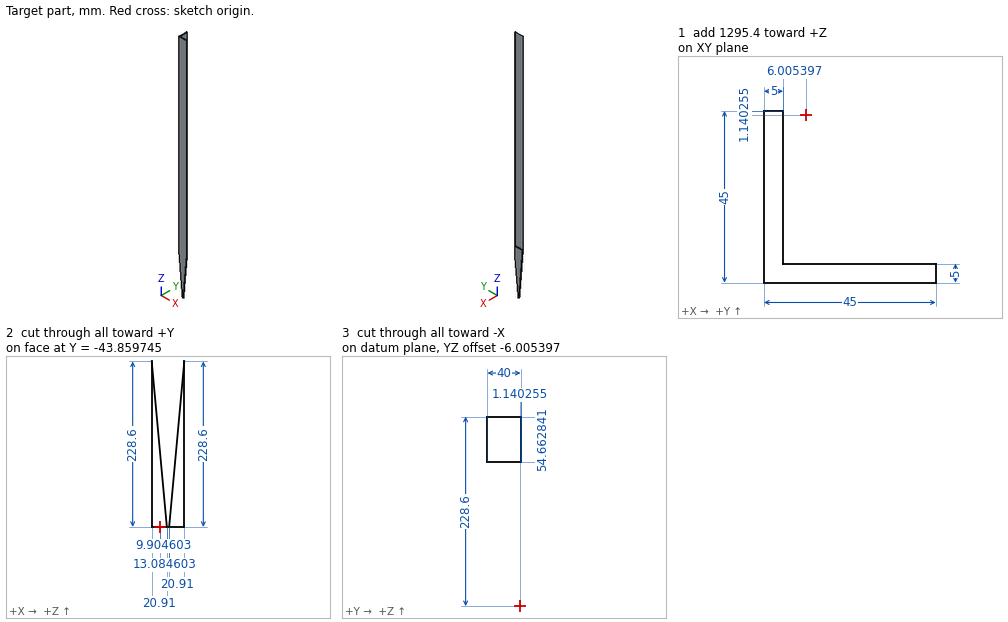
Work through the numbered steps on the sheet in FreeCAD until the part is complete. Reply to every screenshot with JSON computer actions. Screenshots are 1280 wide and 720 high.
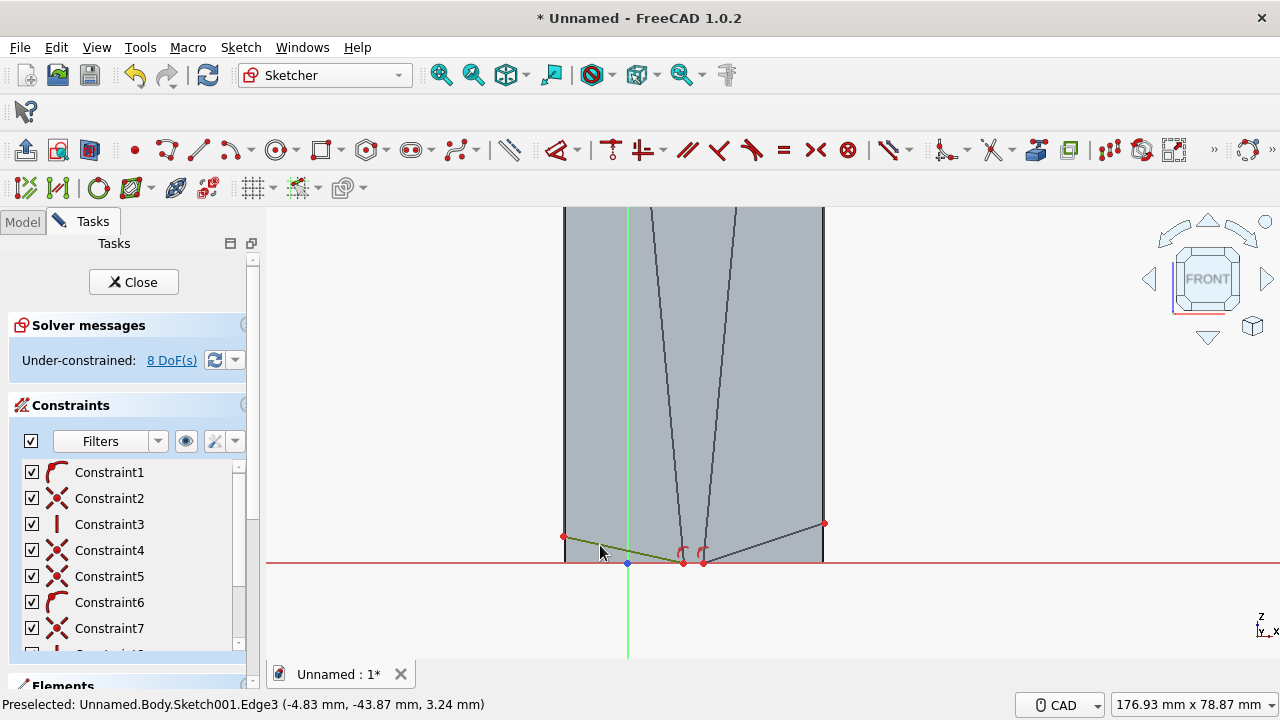
{"action": "key", "text": "h"}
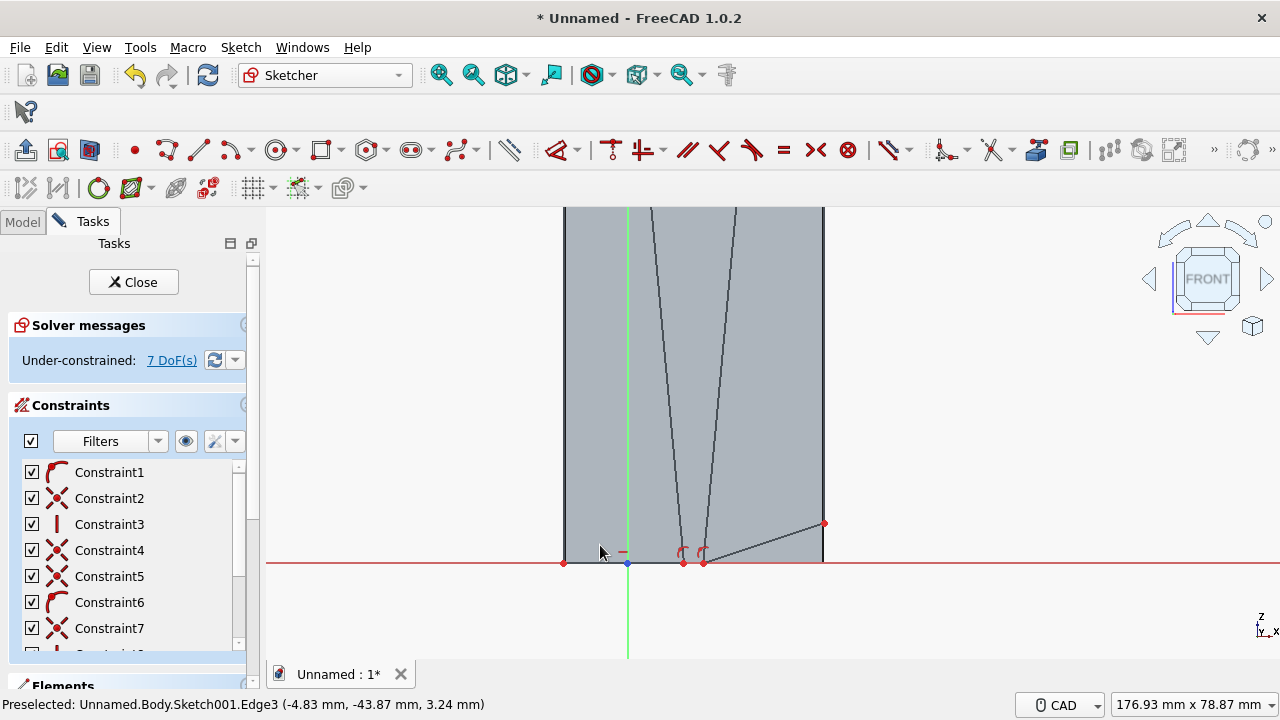
{"action": "left_click", "coordinate": [739, 551]}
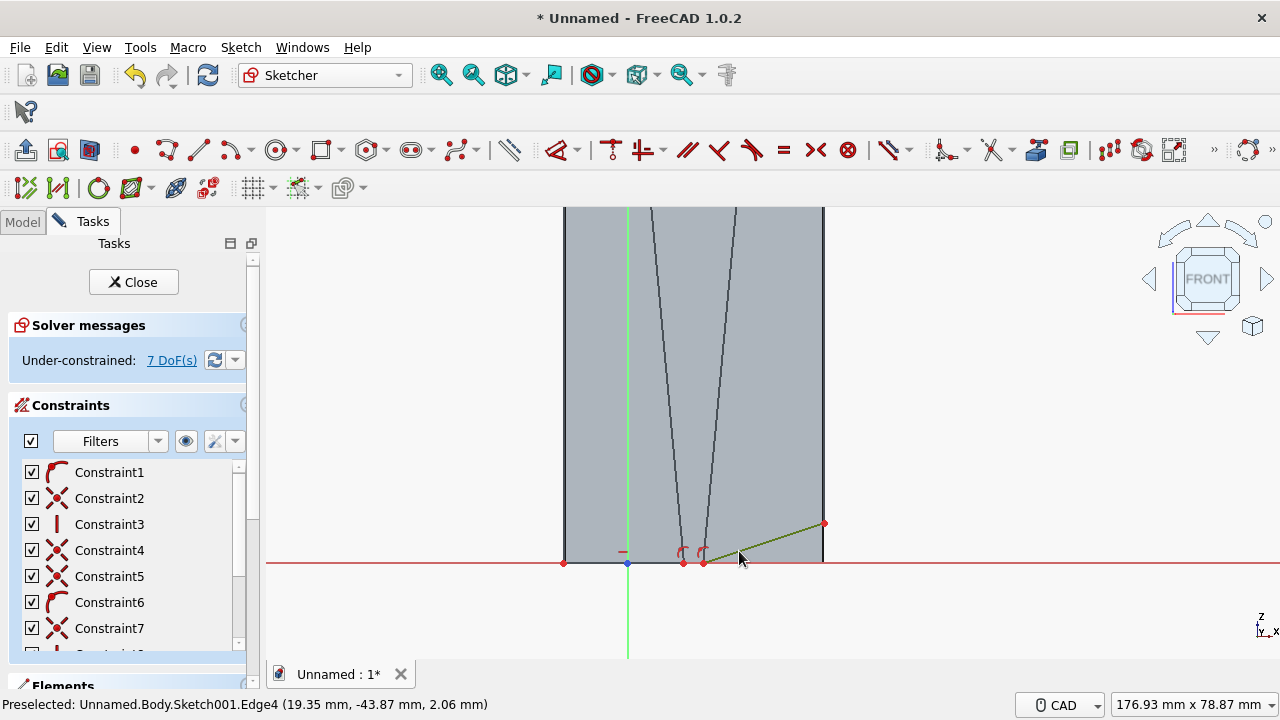
{"action": "key", "text": "h"}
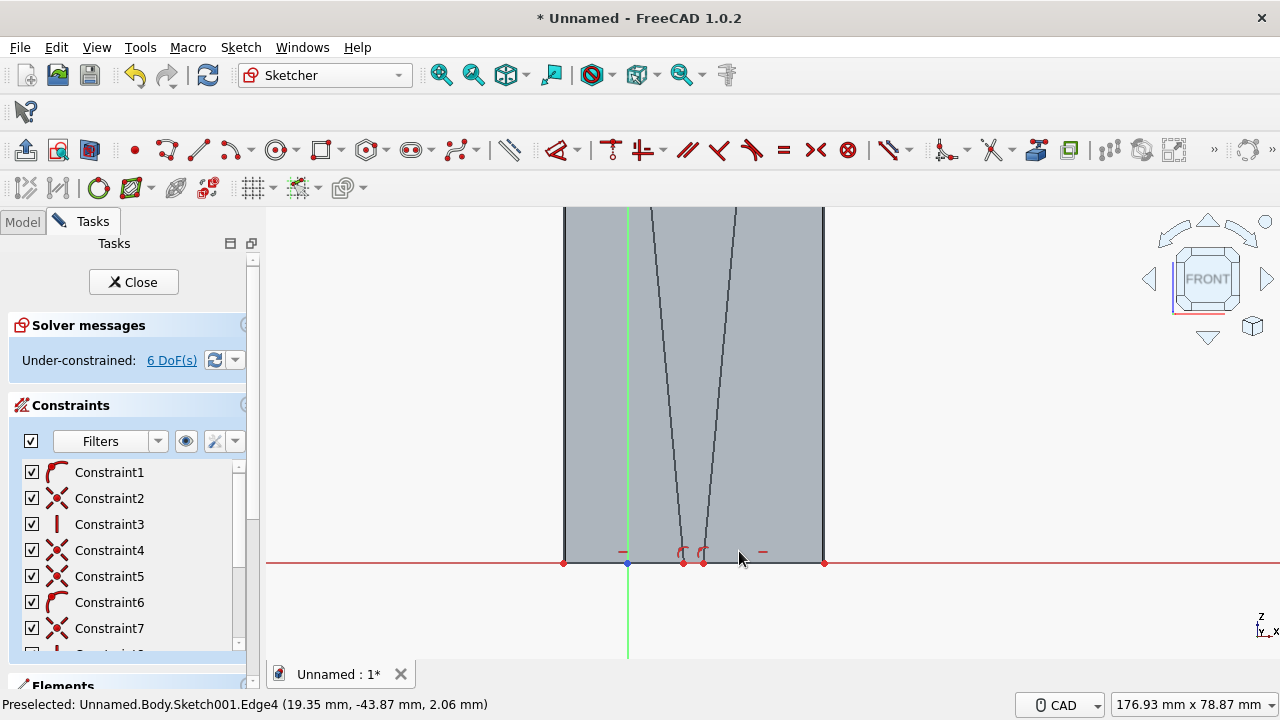
{"action": "left_click", "coordinate": [556, 150]}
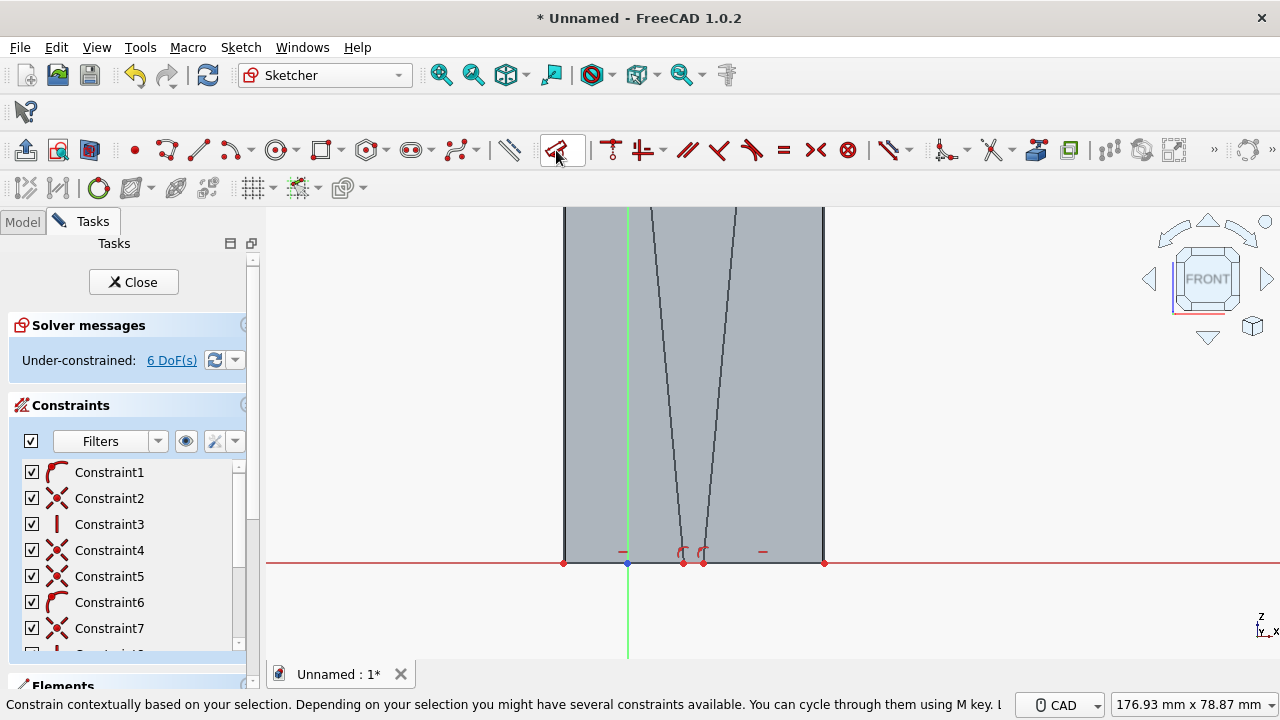
{"action": "scroll", "coordinate": [707, 566], "scroll_direction": "down", "scroll_amount": 8}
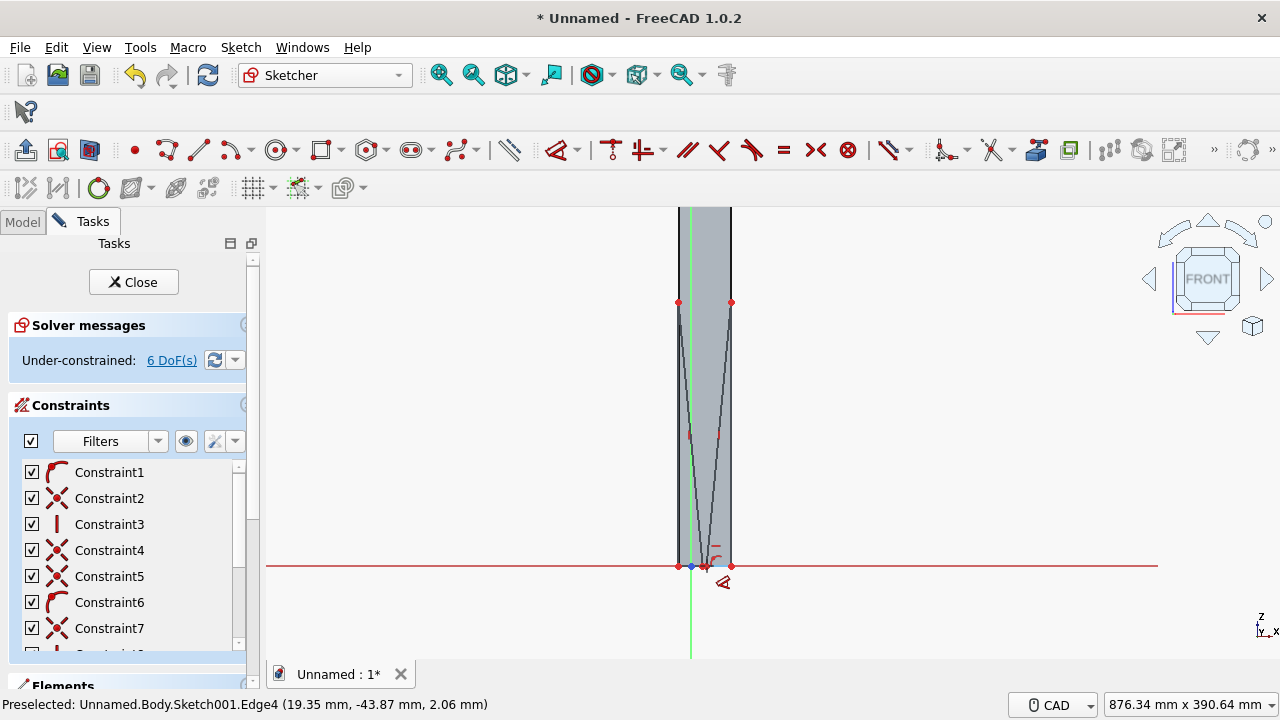
{"action": "left_click", "coordinate": [678, 513]}
{"action": "left_click", "coordinate": [644, 434]}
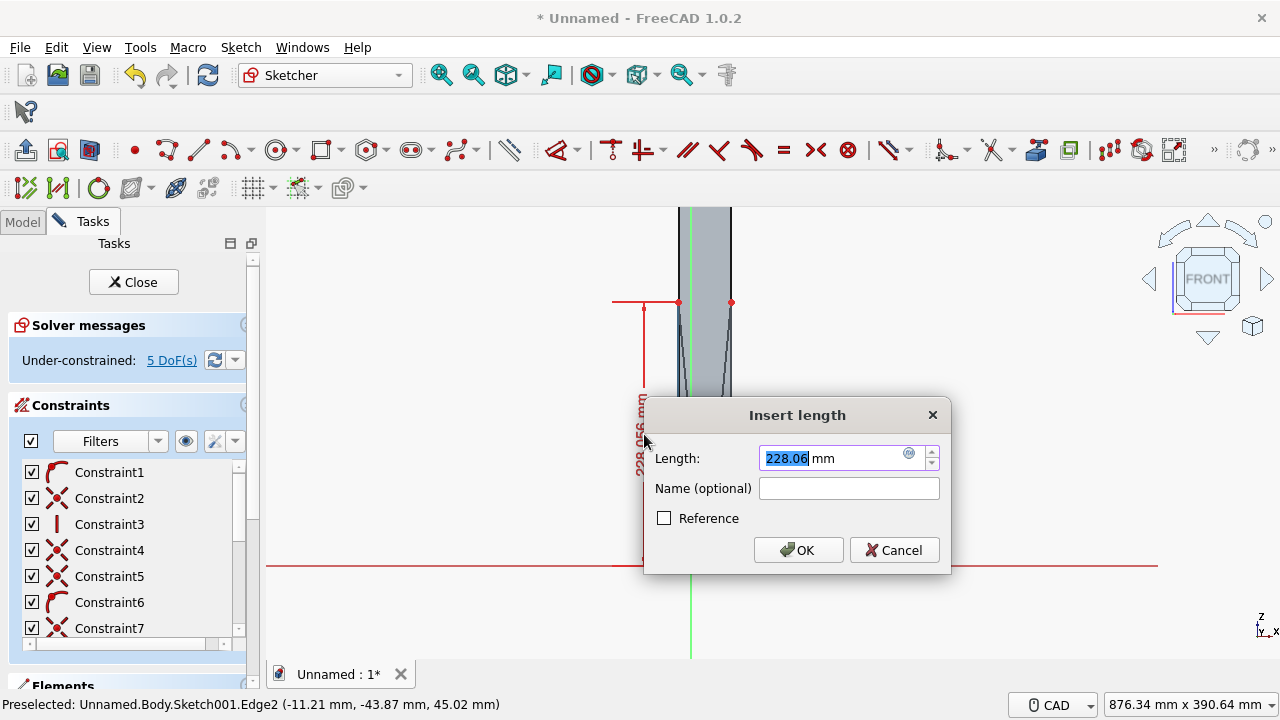
{"action": "type", "text": "228.6"}
{"action": "key", "text": "Return"}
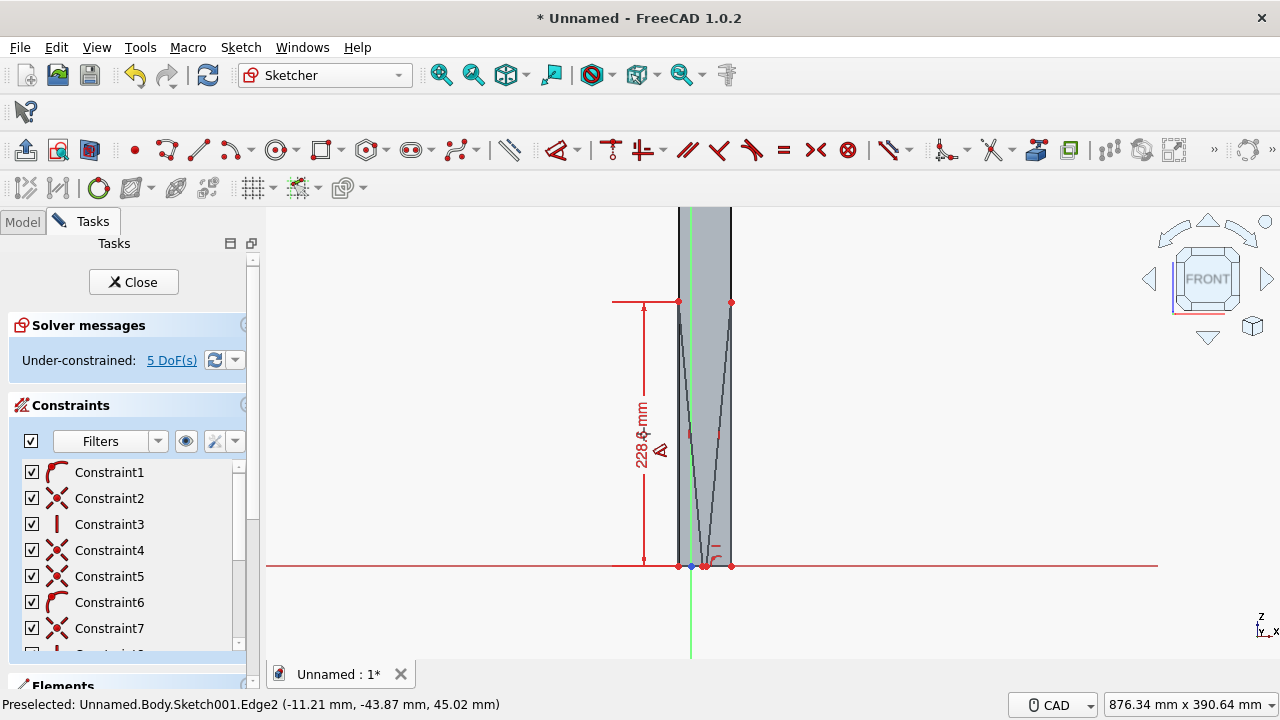
{"action": "scroll", "coordinate": [688, 566], "scroll_direction": "up", "scroll_amount": 3}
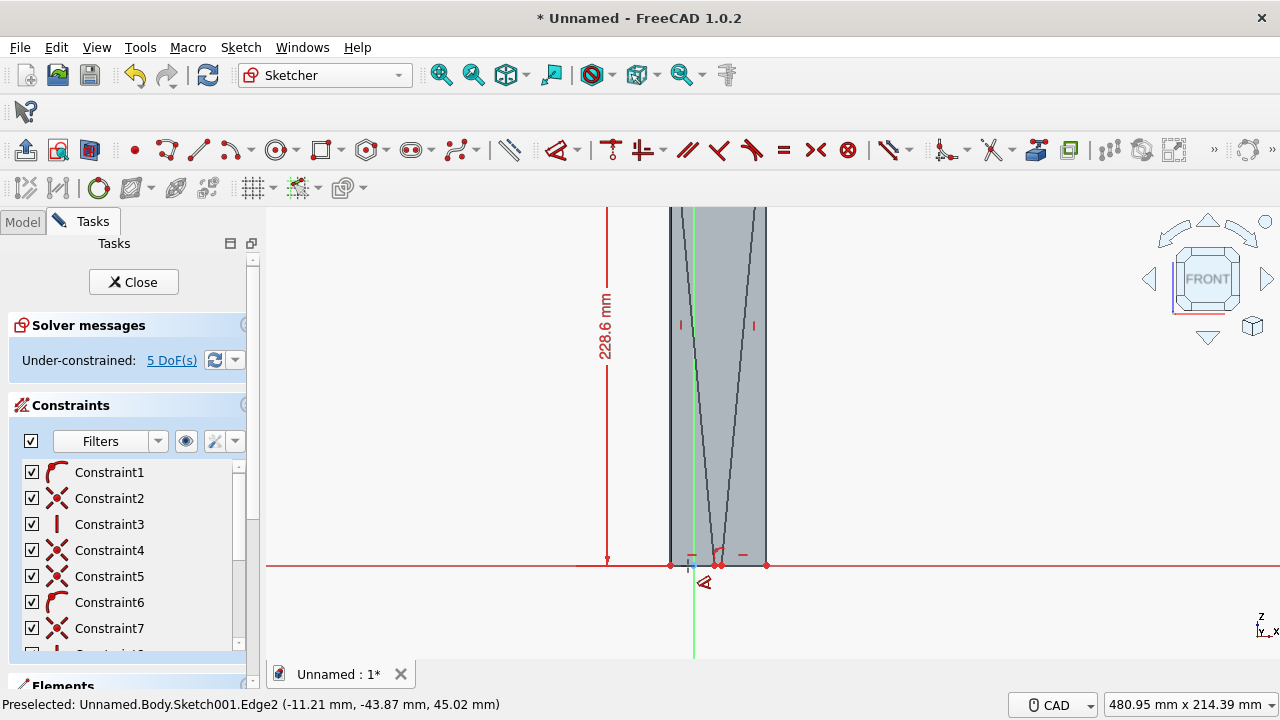
{"action": "left_click", "coordinate": [688, 566]}
{"action": "left_click", "coordinate": [677, 600]}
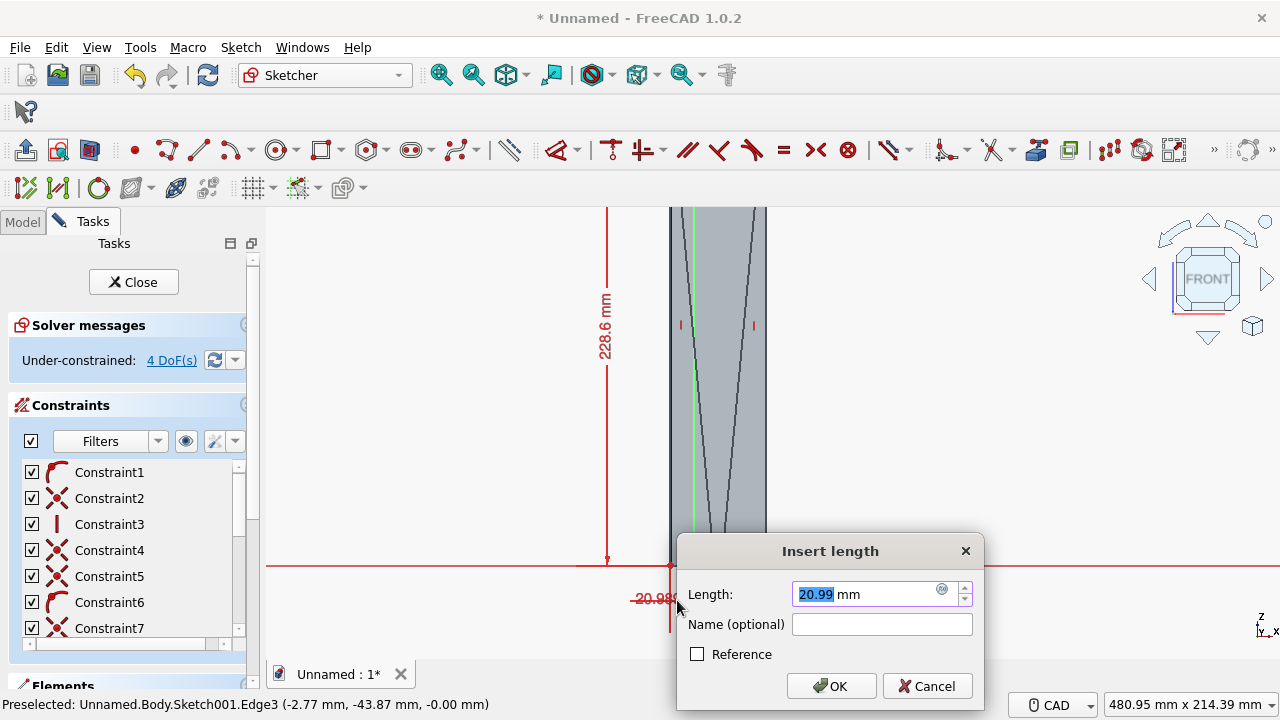
{"action": "type", "text": "20.91"}
{"action": "key", "text": "Return"}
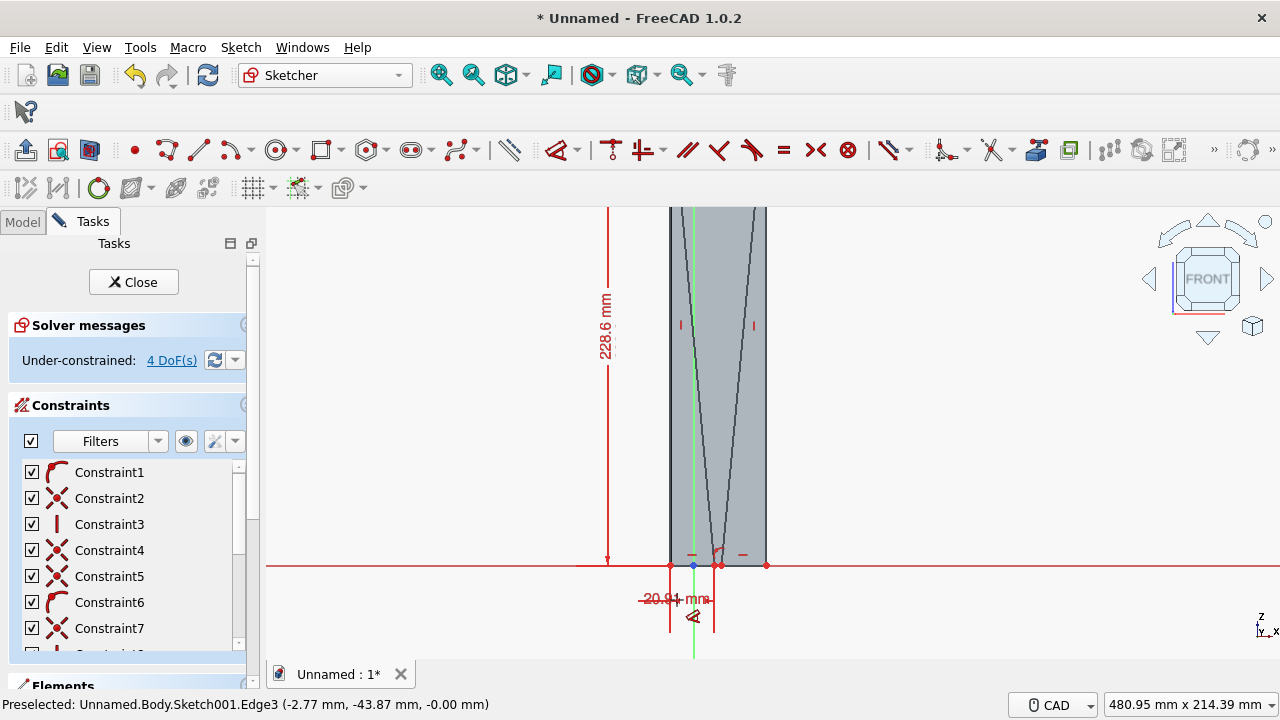
{"action": "left_click", "coordinate": [735, 566]}
{"action": "left_click", "coordinate": [754, 600]}